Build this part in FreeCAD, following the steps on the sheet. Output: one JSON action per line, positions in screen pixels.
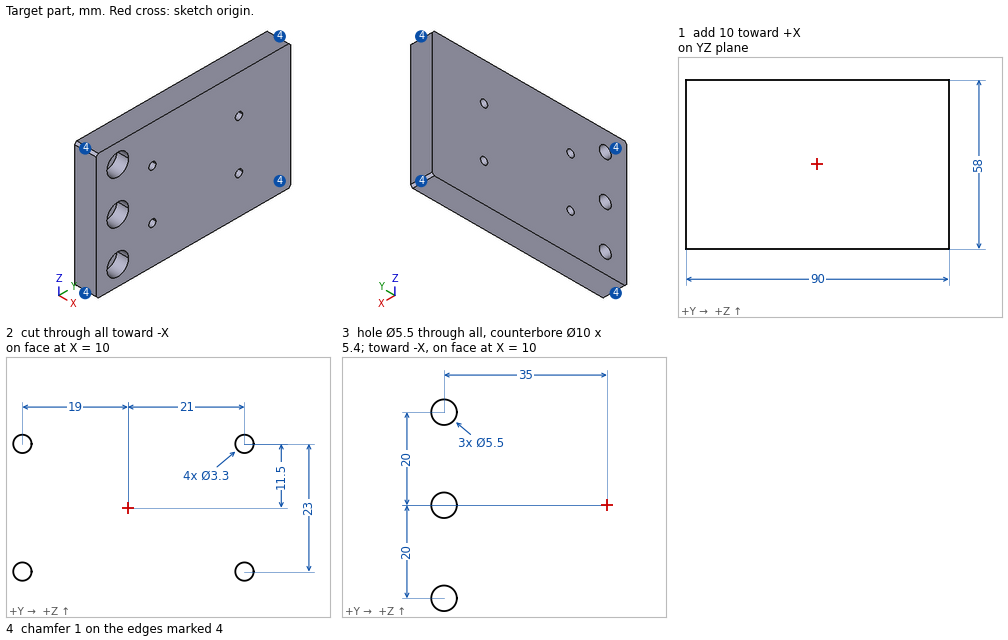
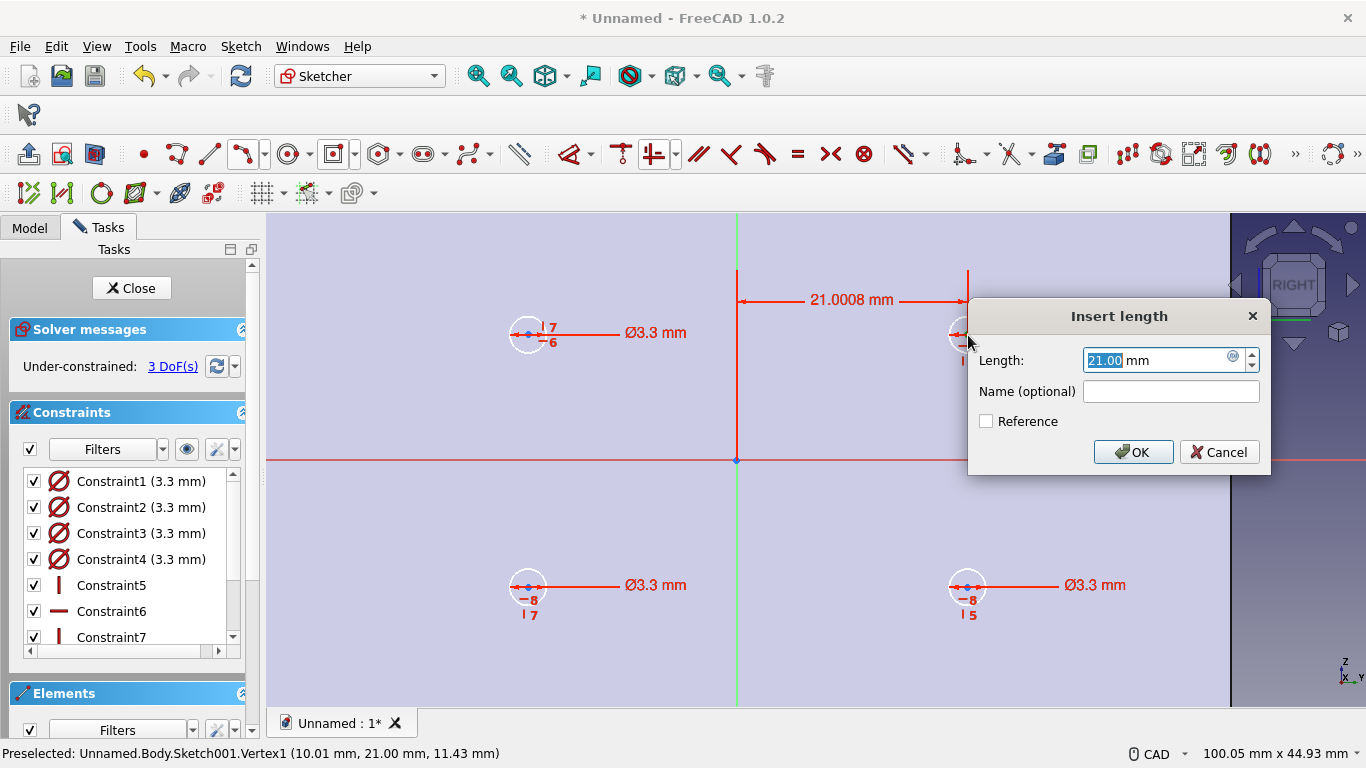
{"action": "type", "text": "21"}
{"action": "key", "text": "Return"}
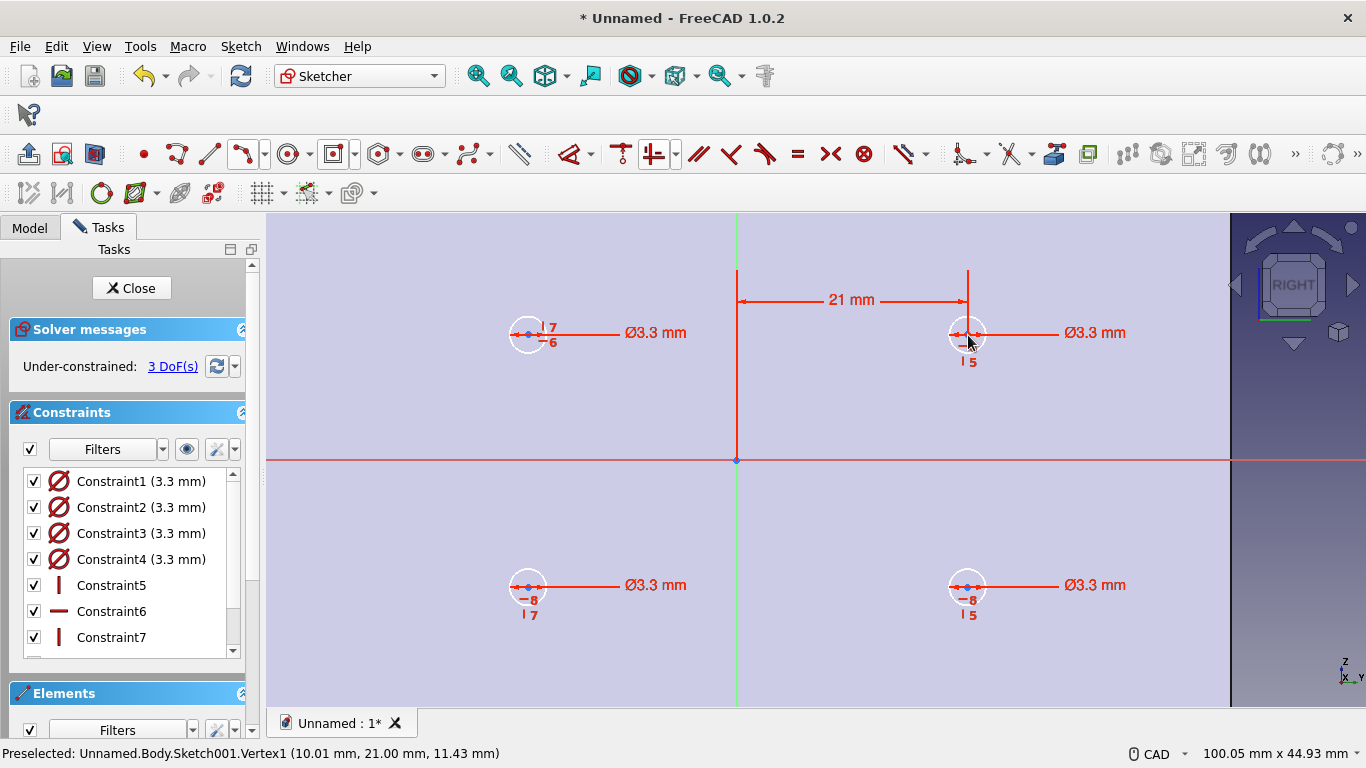
{"action": "left_click", "coordinate": [528, 335]}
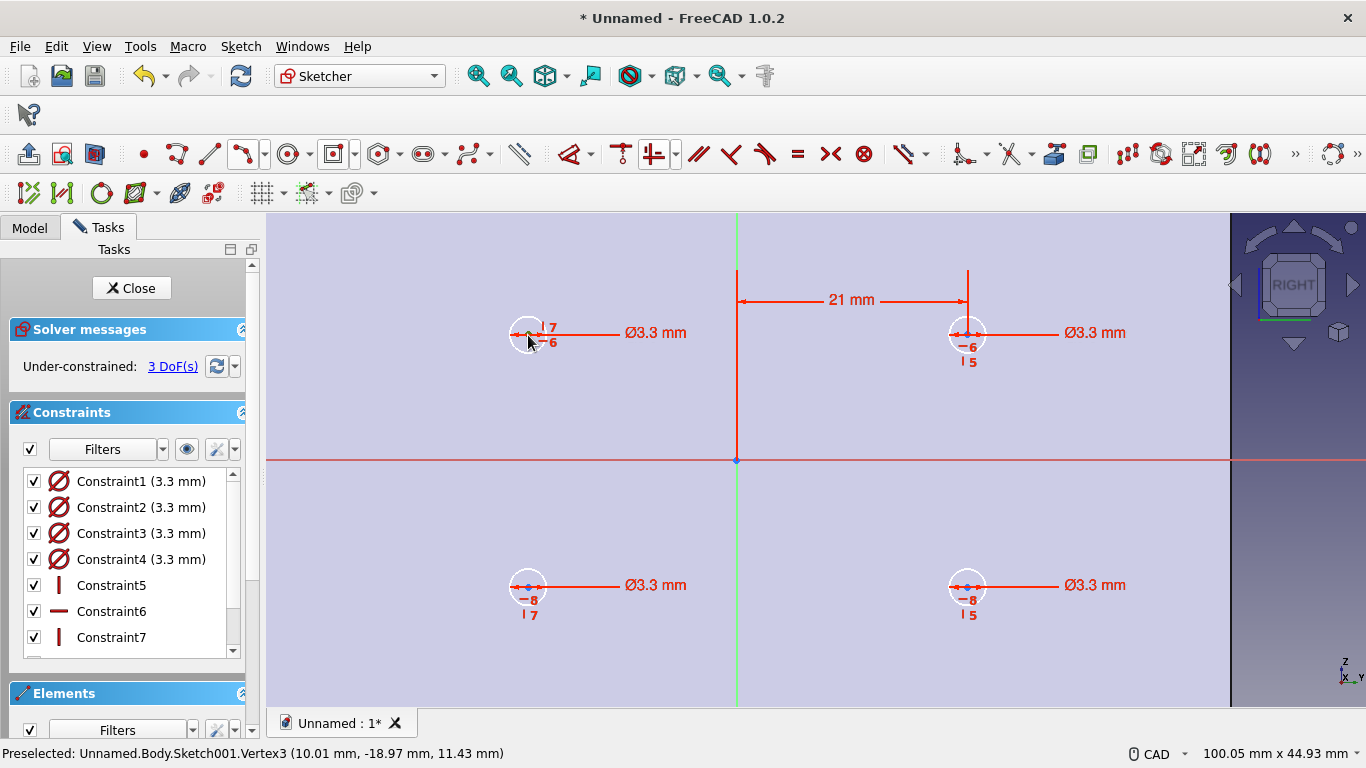
{"action": "left_click", "coordinate": [590, 154]}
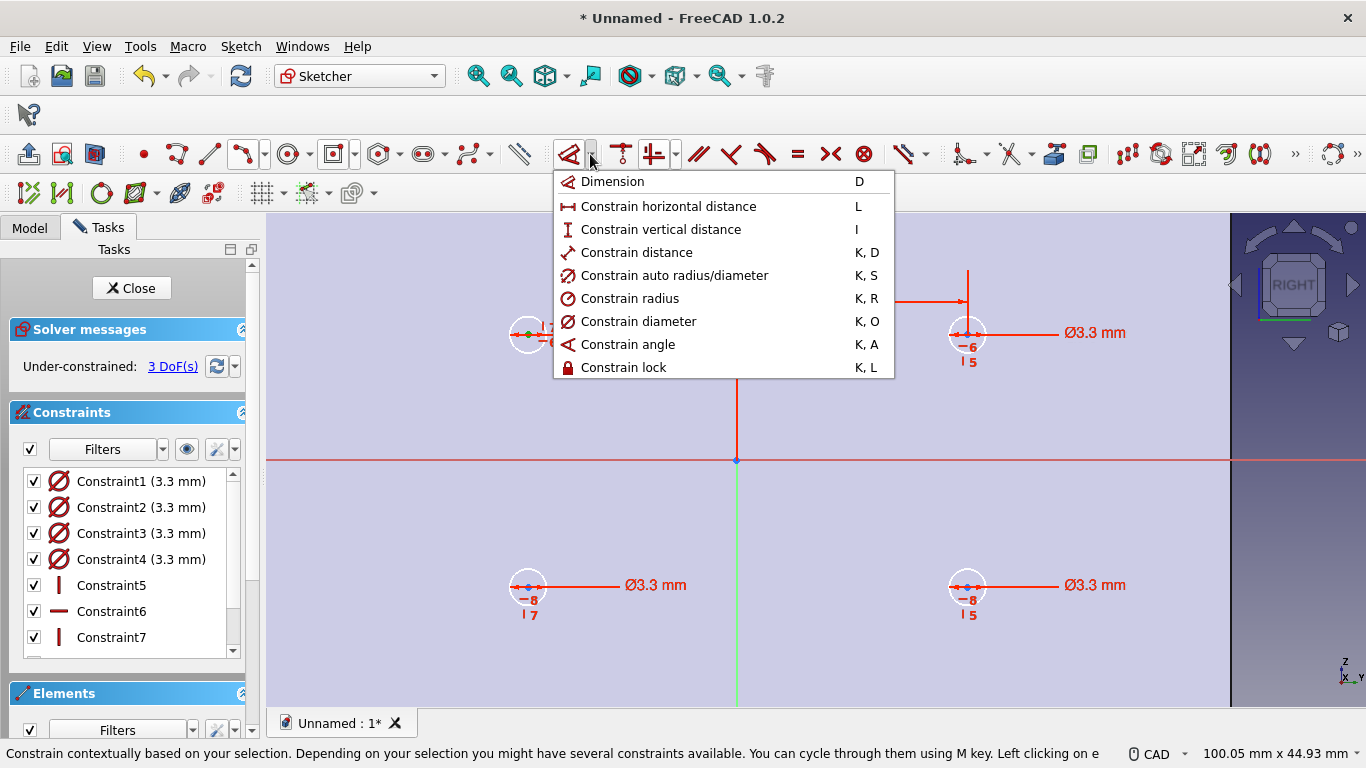
{"action": "left_click", "coordinate": [724, 206]}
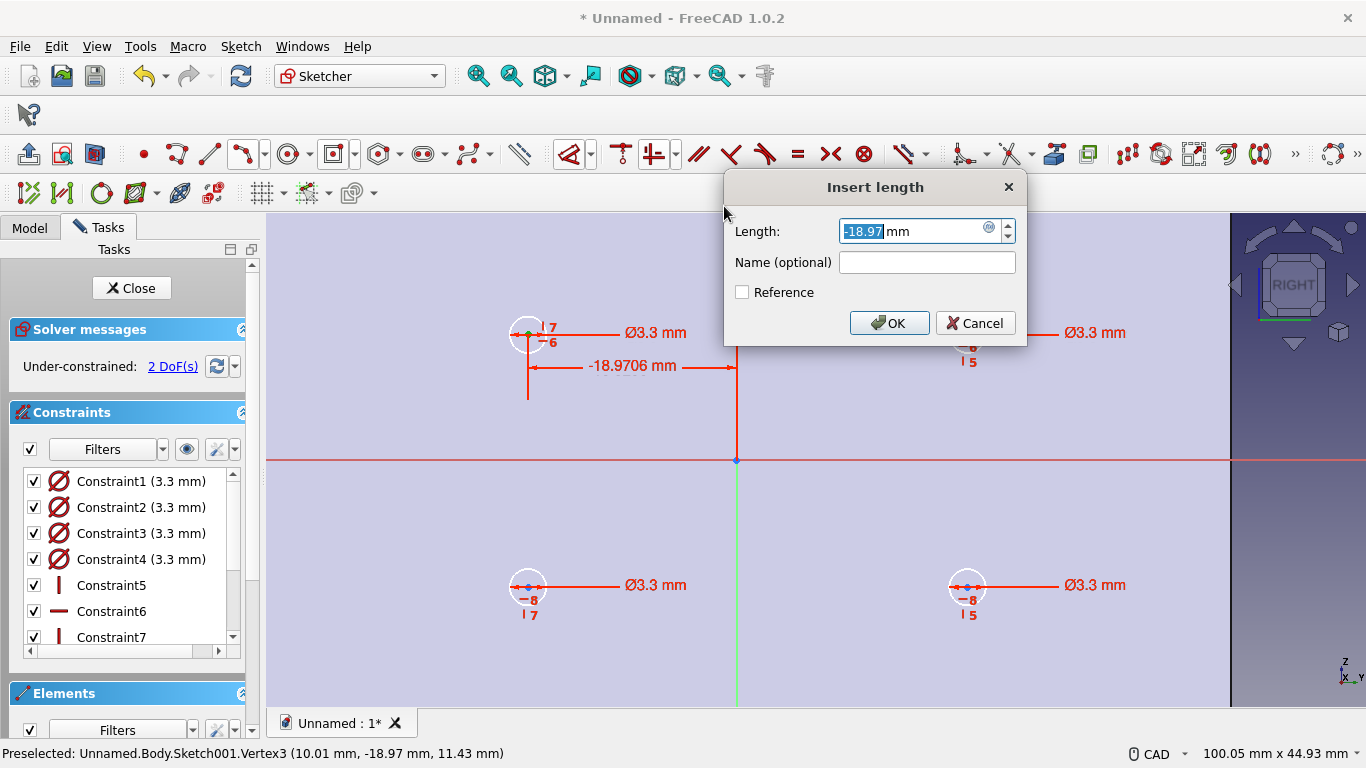
{"action": "type", "text": "-19"}
{"action": "key", "text": "Return"}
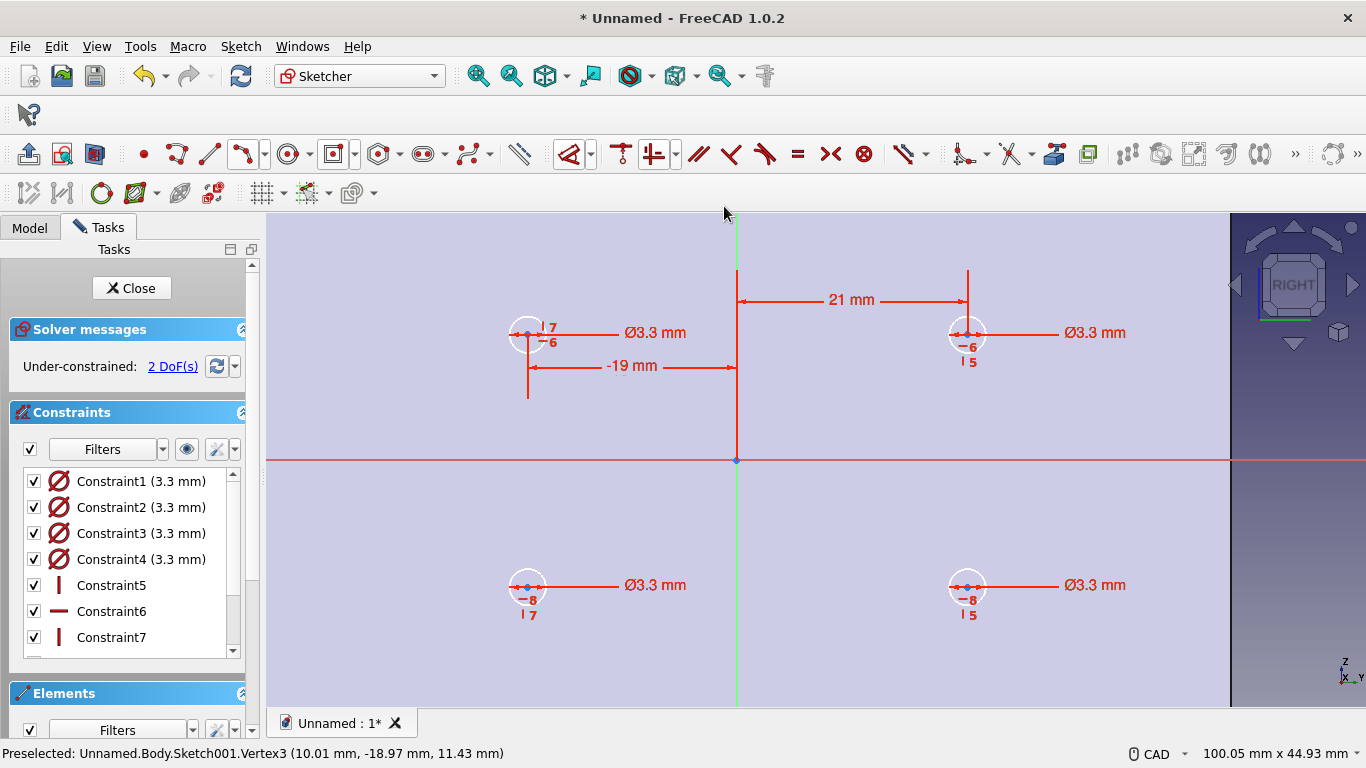
{"action": "left_click", "coordinate": [968, 335]}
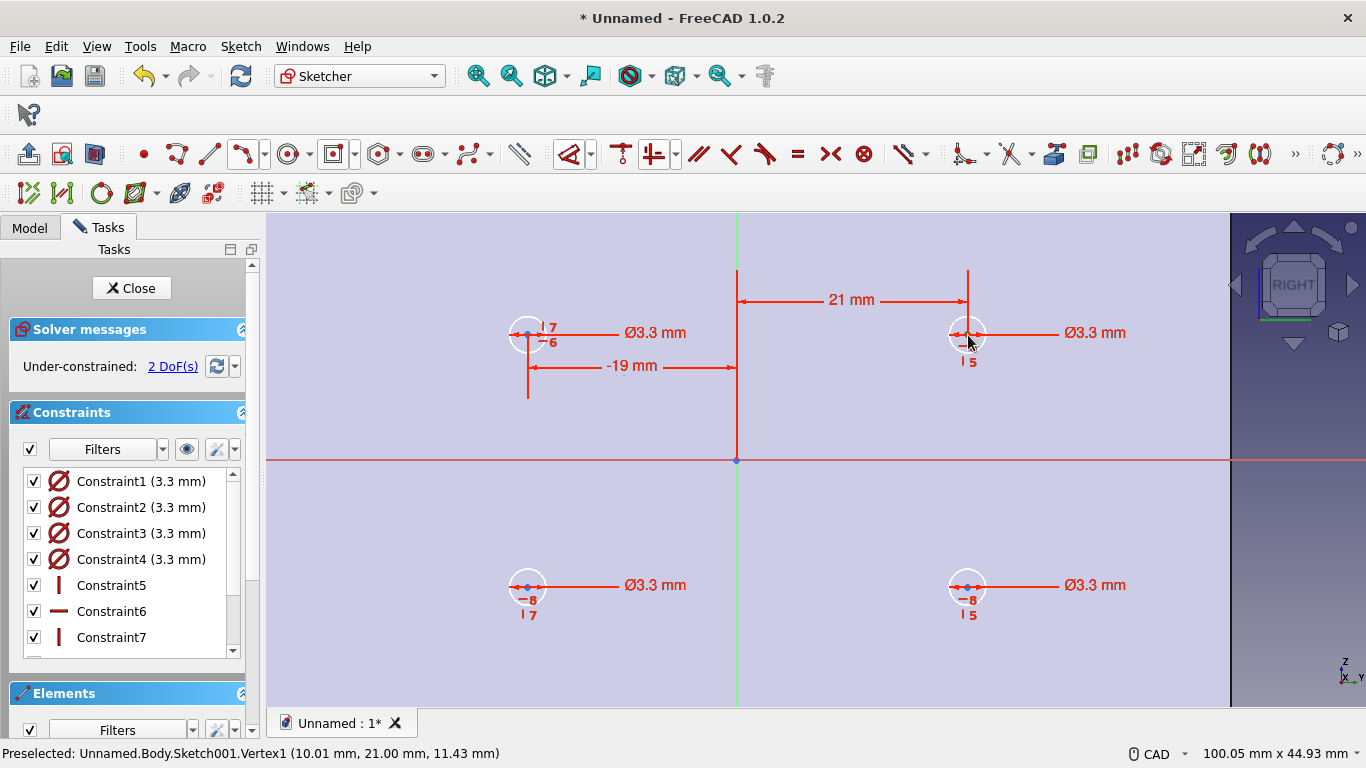
{"action": "left_click", "coordinate": [968, 587]}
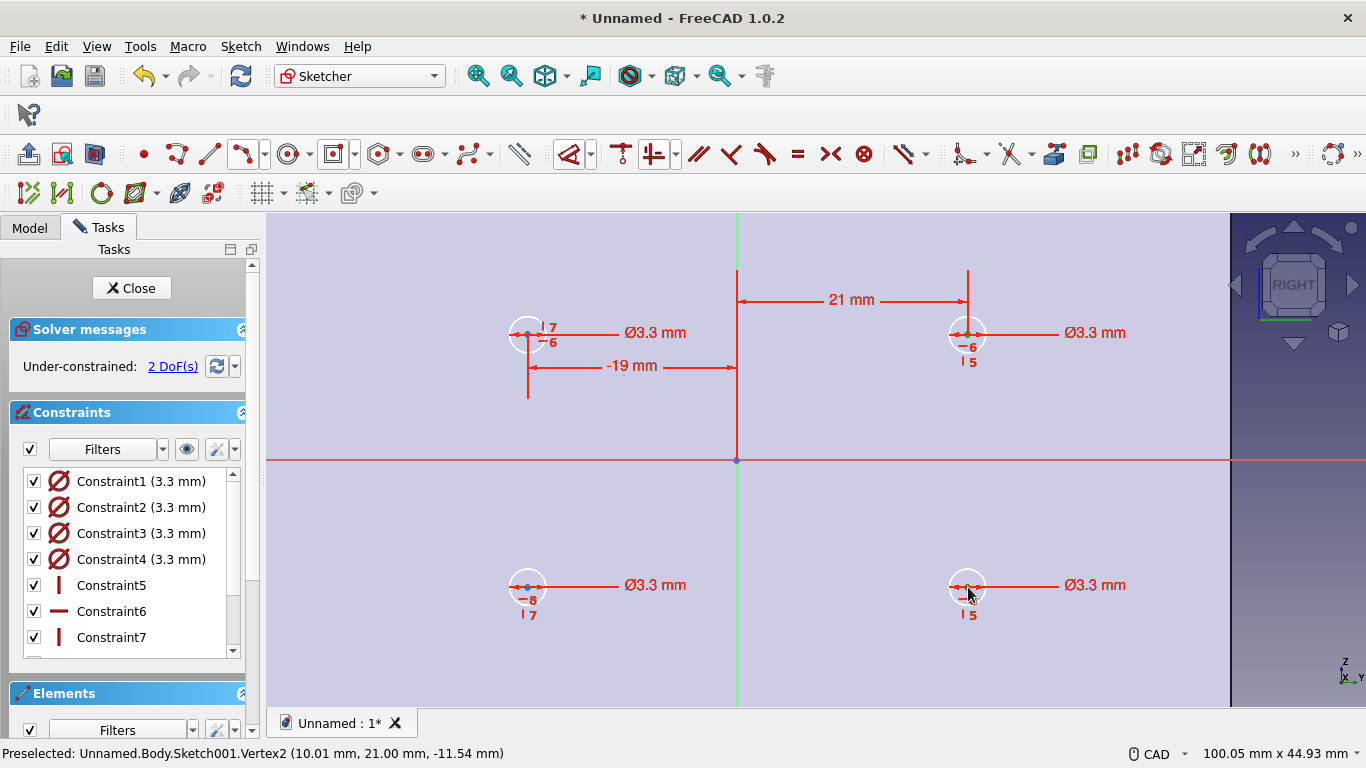
{"action": "key", "text": "i"}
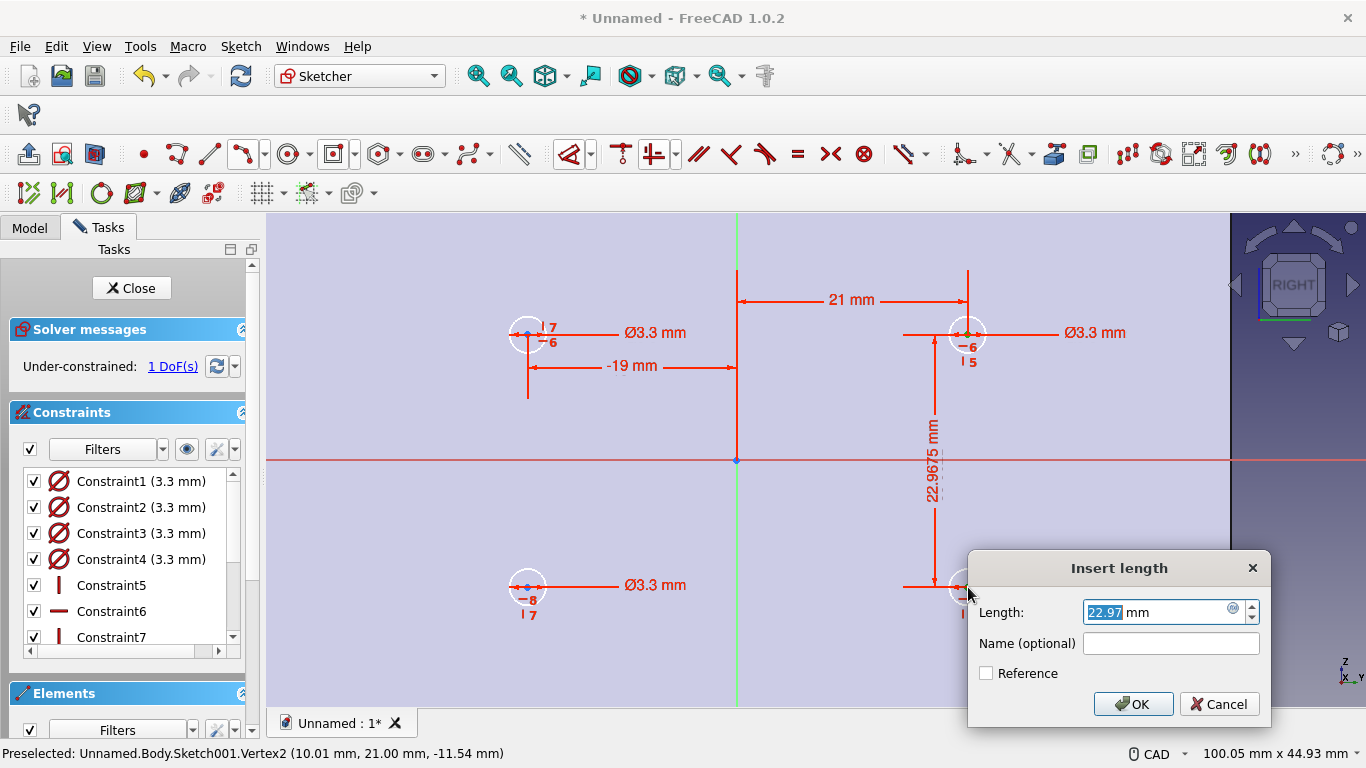
{"action": "type", "text": "23"}
{"action": "key", "text": "Return"}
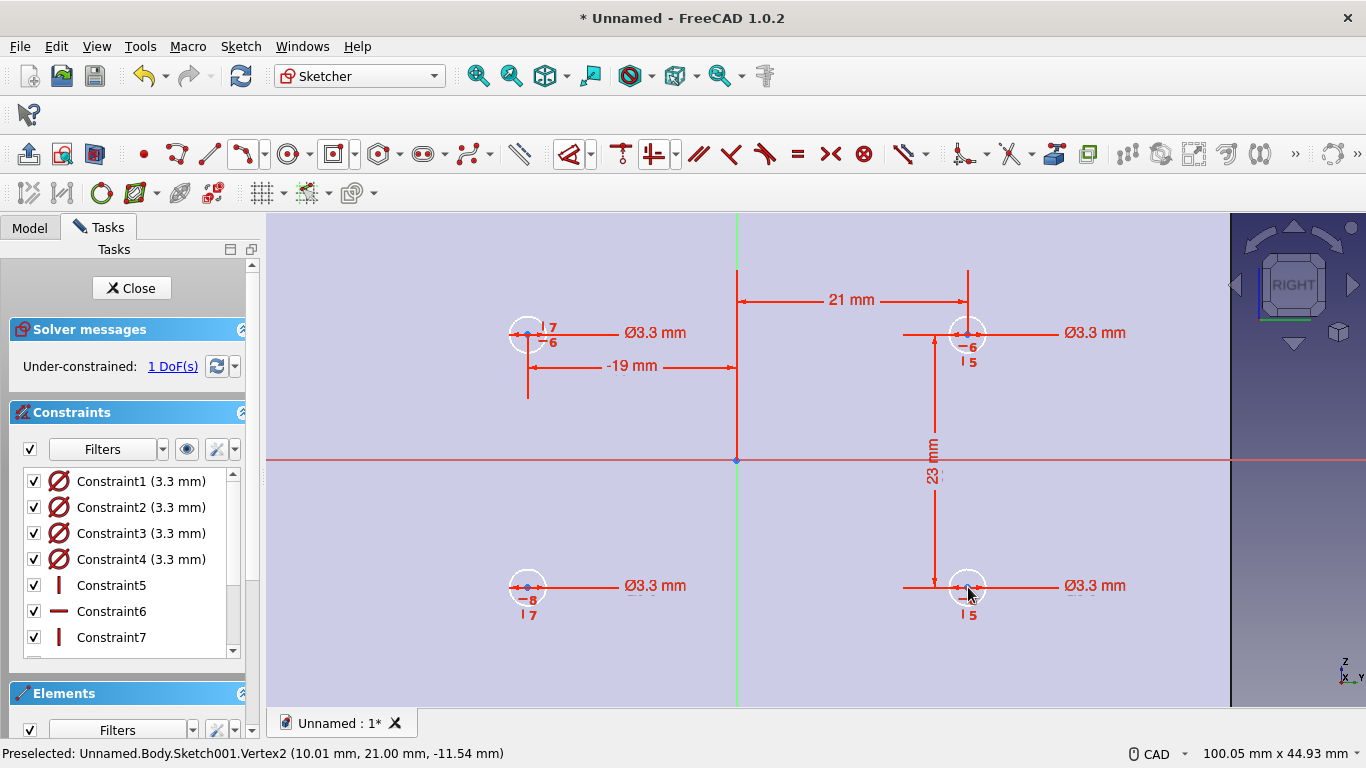
{"action": "left_click", "coordinate": [968, 335]}